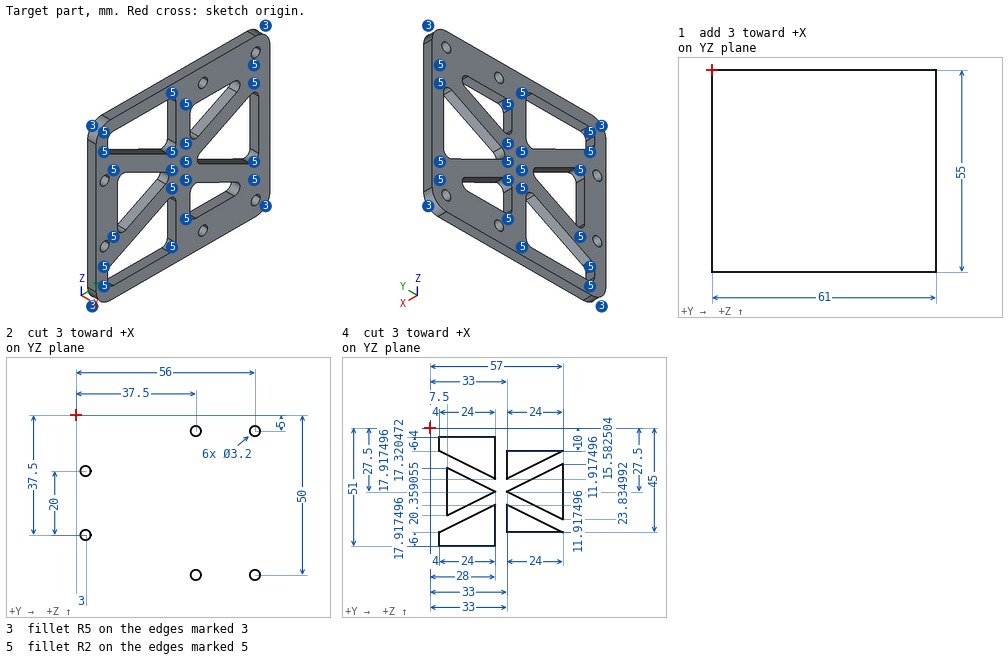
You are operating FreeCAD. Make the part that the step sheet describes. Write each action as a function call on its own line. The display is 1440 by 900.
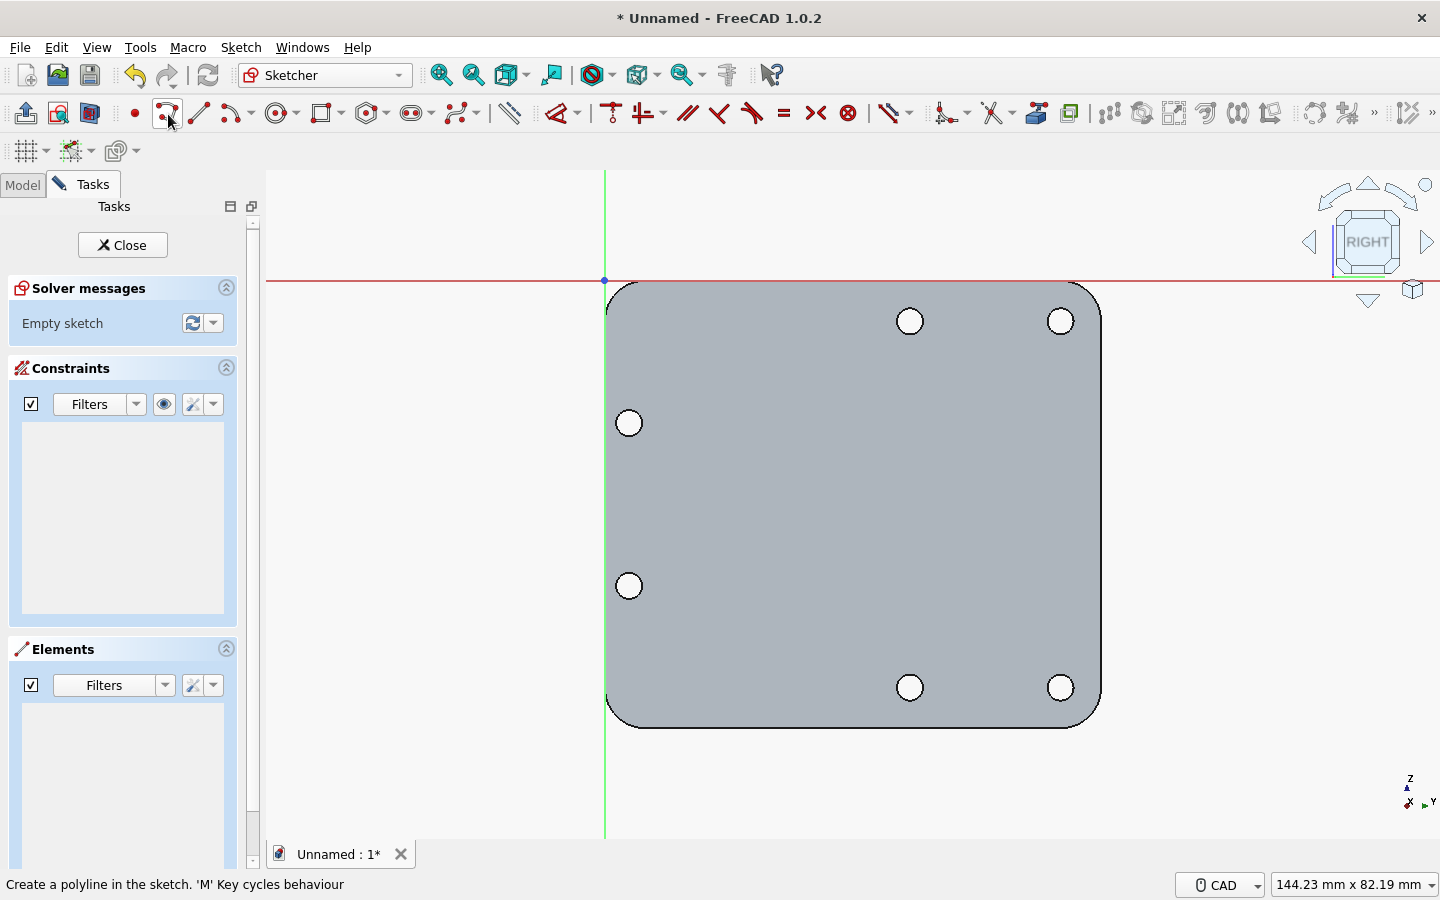
click(873, 504)
click(1069, 407)
click(1069, 602)
click(873, 505)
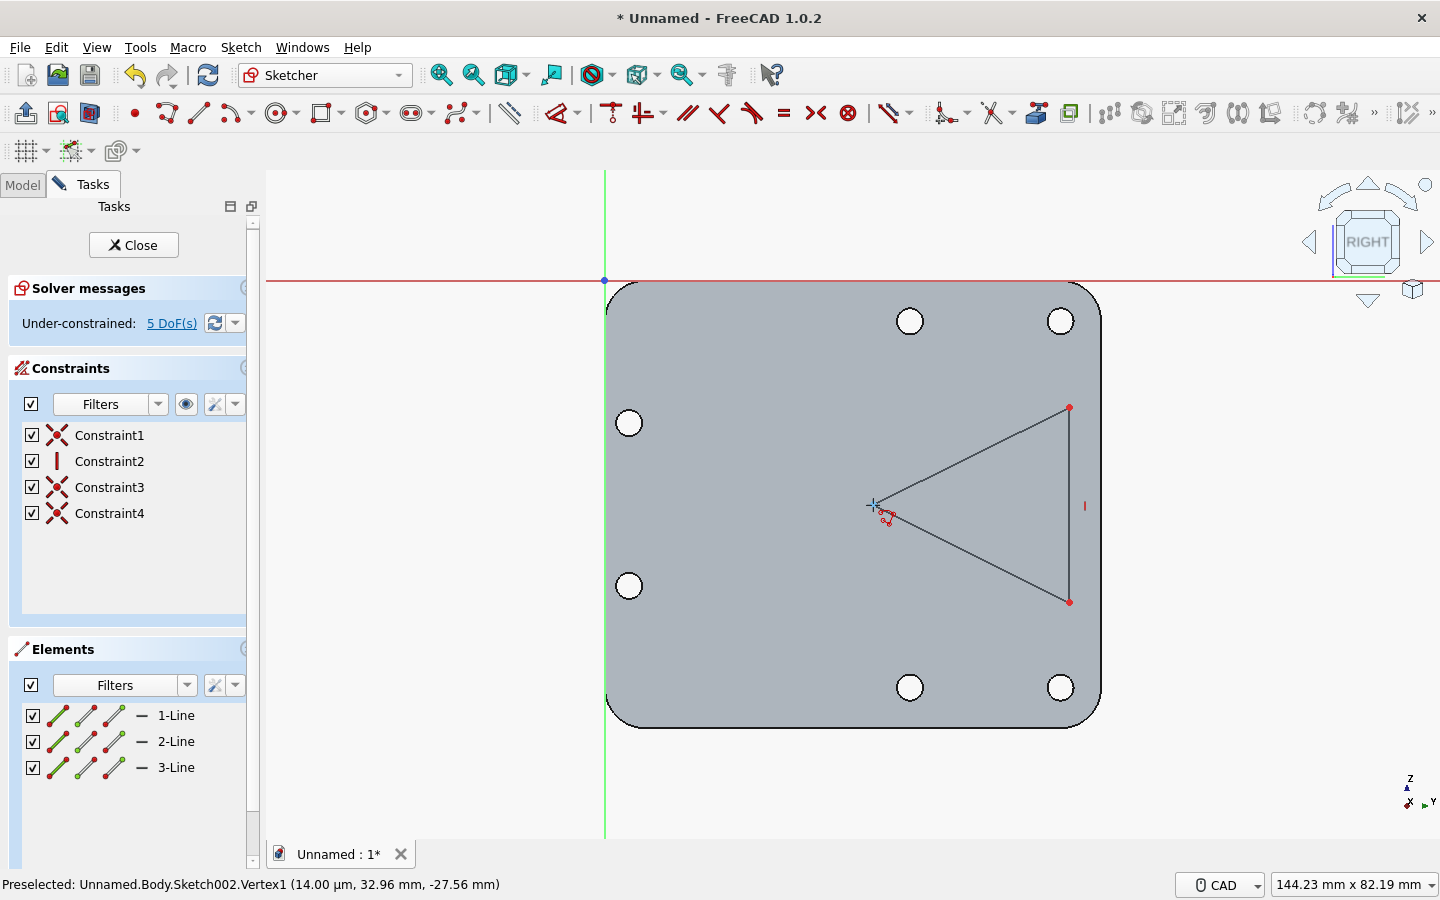
click(873, 550)
click(1069, 647)
click(873, 647)
click(873, 551)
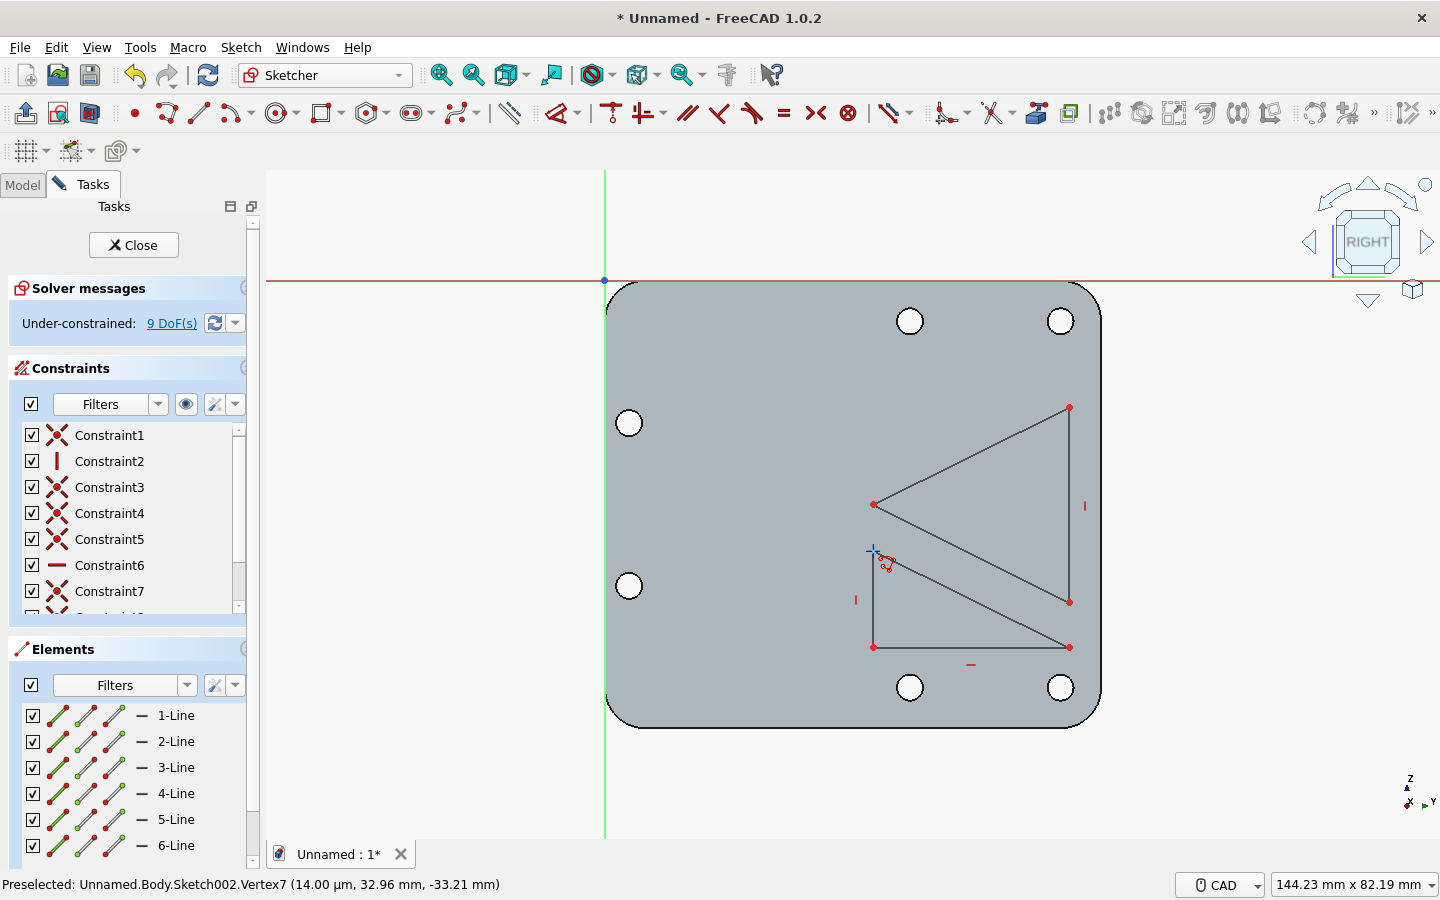
click(873, 362)
click(1069, 362)
click(873, 459)
click(873, 363)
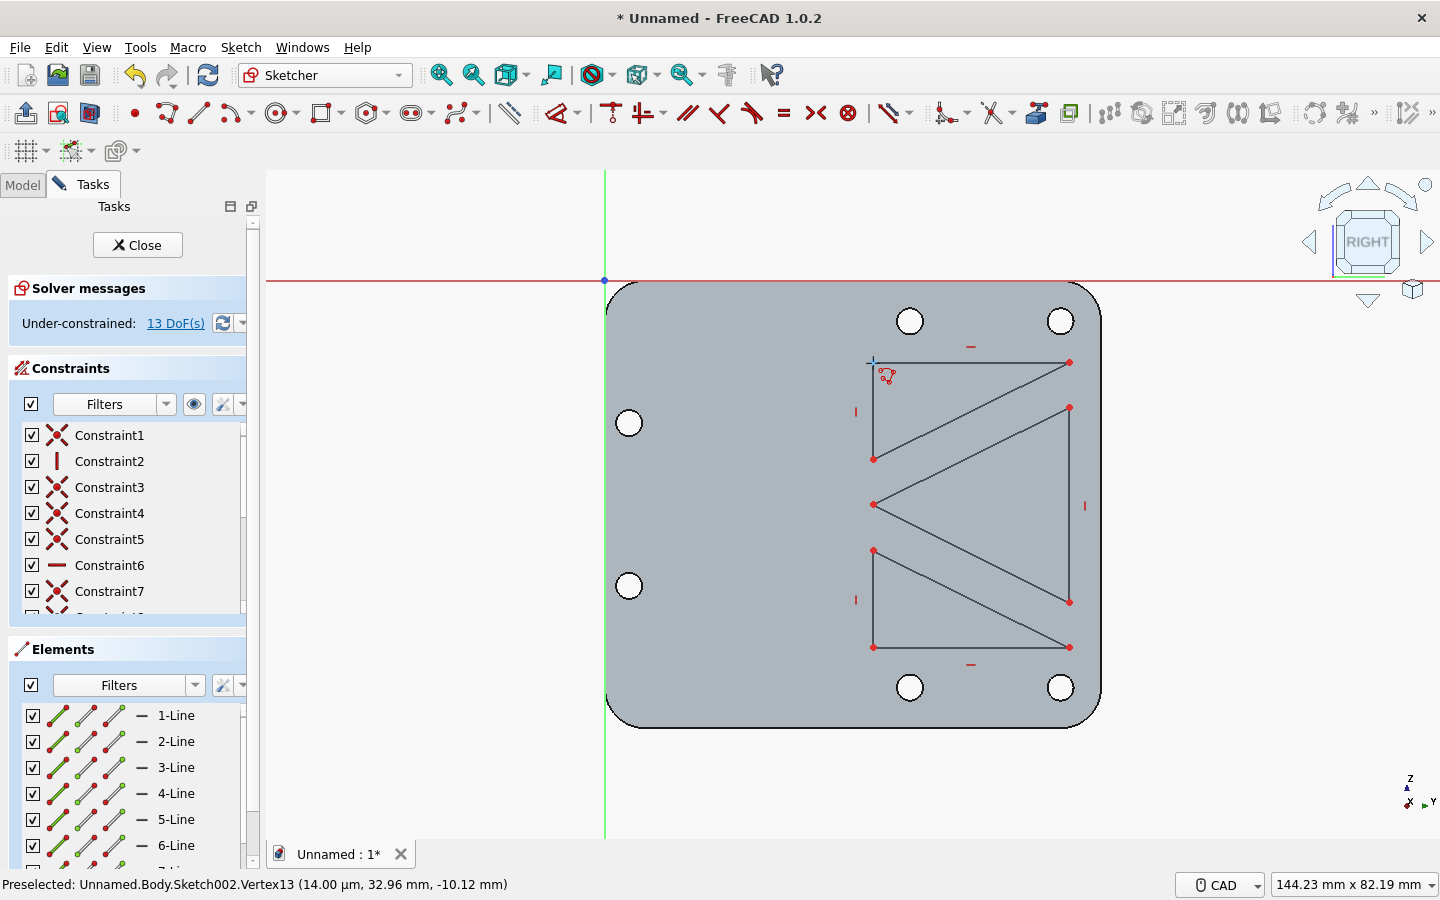
click(637, 313)
click(833, 313)
click(833, 459)
click(637, 362)
click(637, 314)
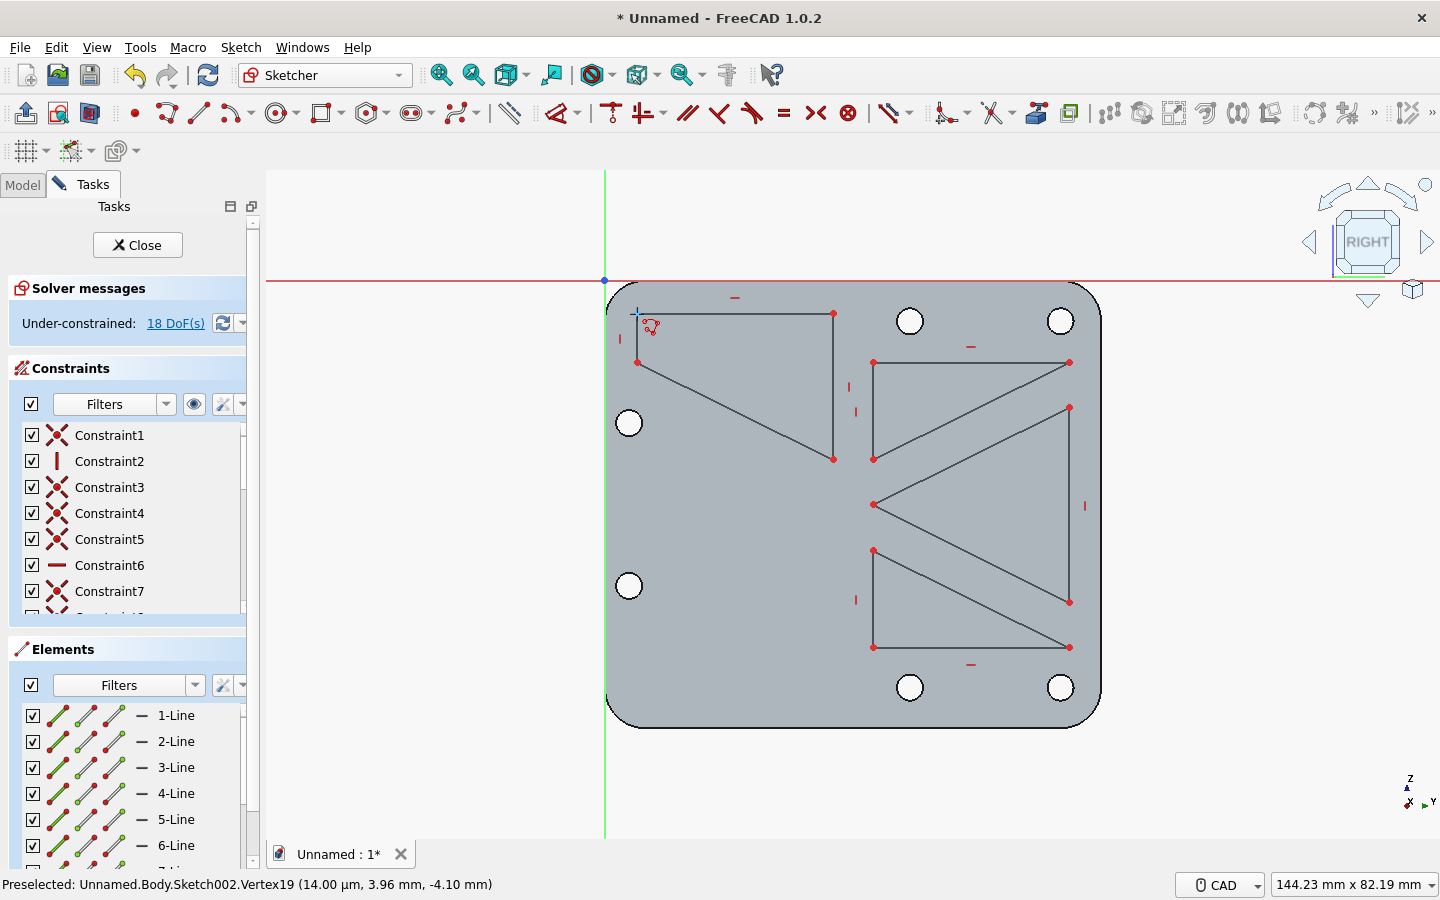
click(666, 422)
click(833, 504)
click(666, 587)
click(666, 423)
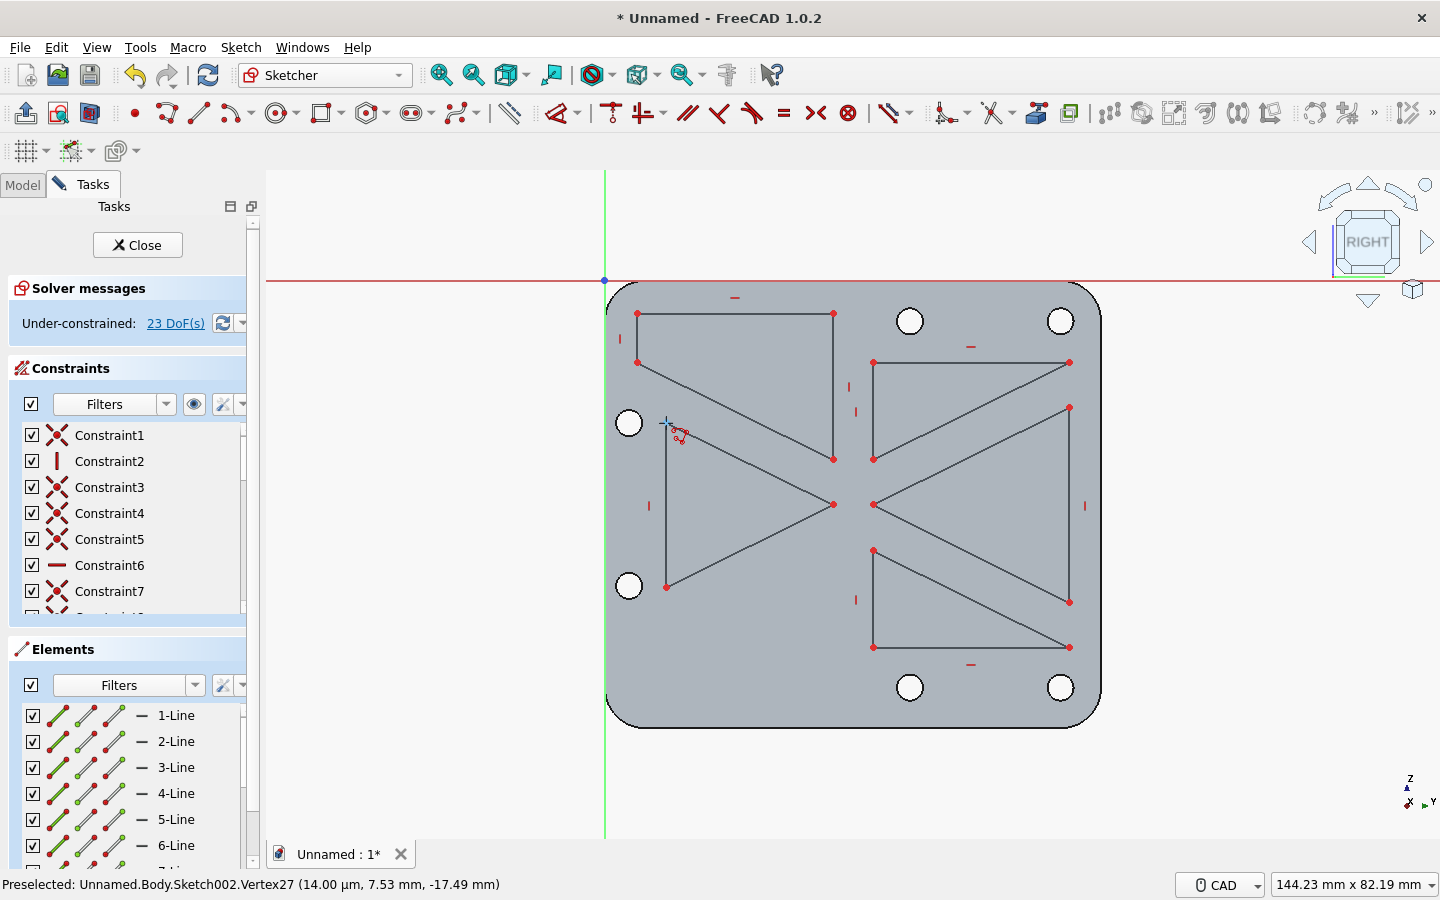
click(833, 550)
click(833, 696)
click(637, 696)
click(637, 647)
click(833, 551)
key(Escape)
key(Escape)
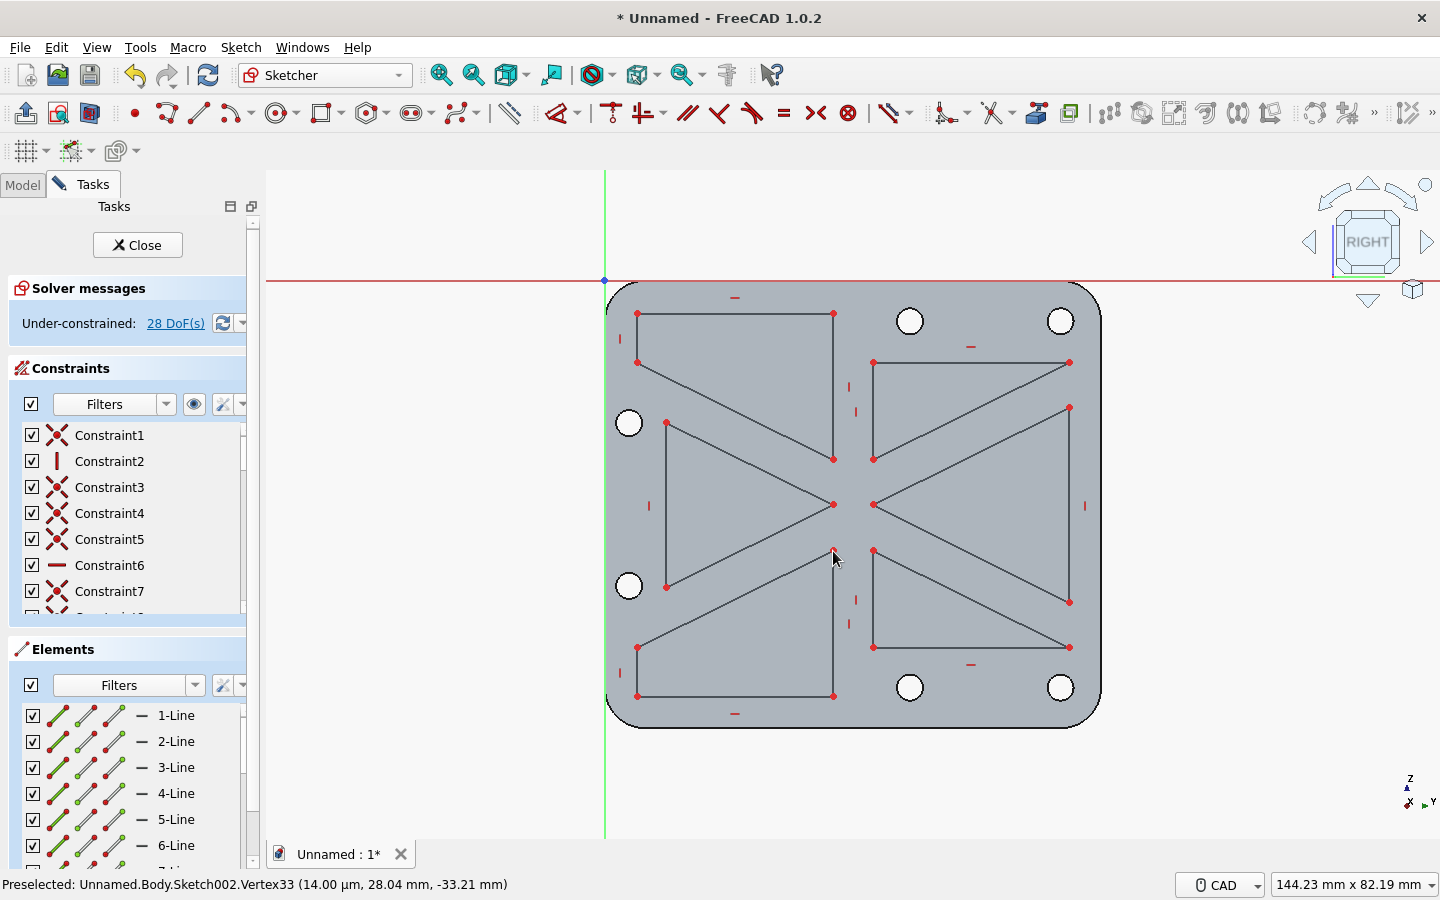
click(556, 114)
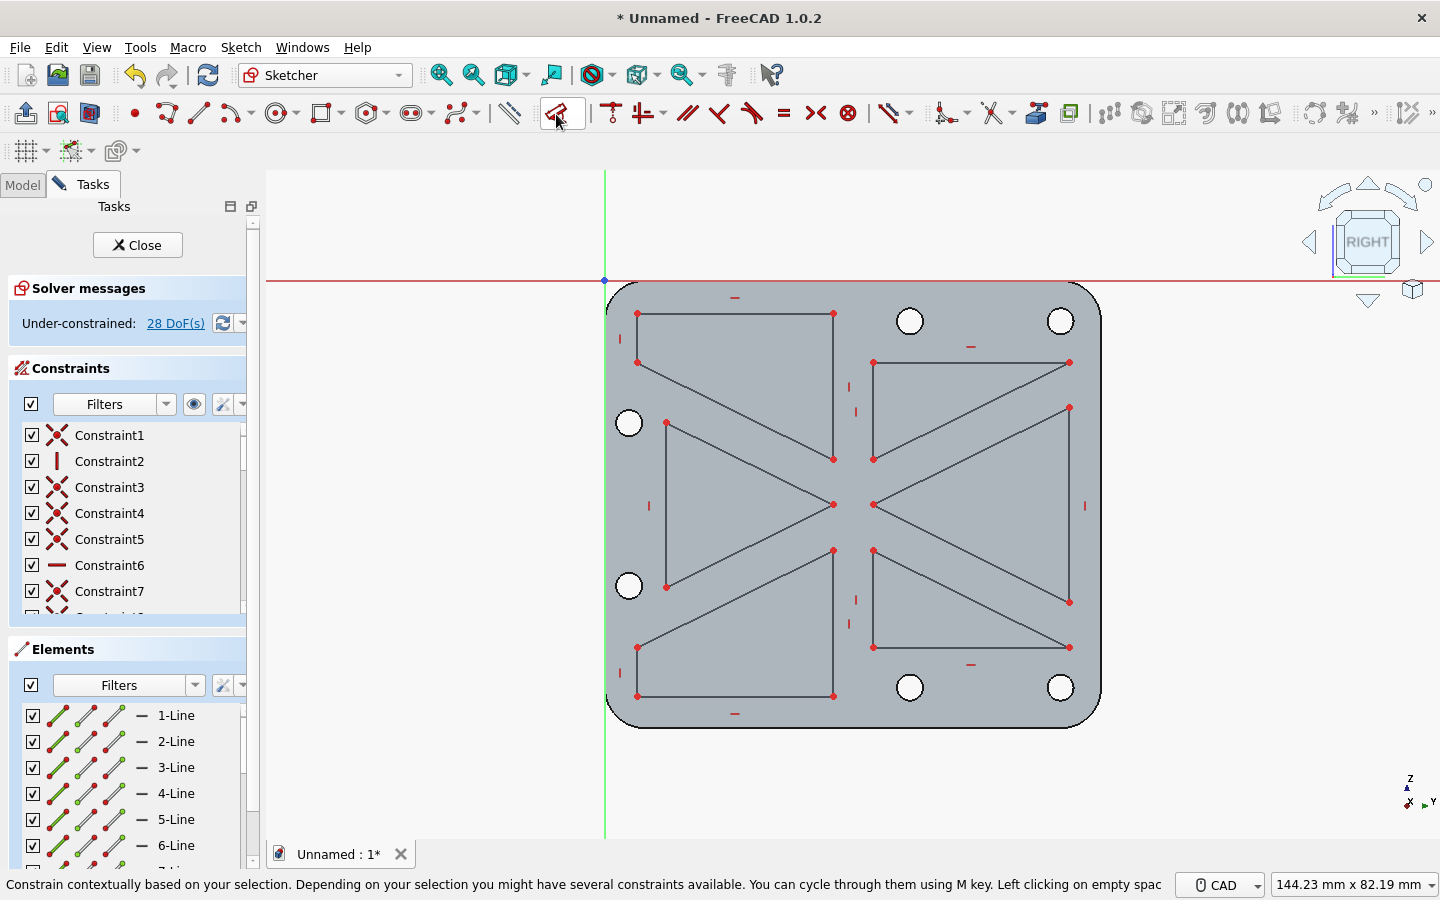
click(637, 348)
click(671, 338)